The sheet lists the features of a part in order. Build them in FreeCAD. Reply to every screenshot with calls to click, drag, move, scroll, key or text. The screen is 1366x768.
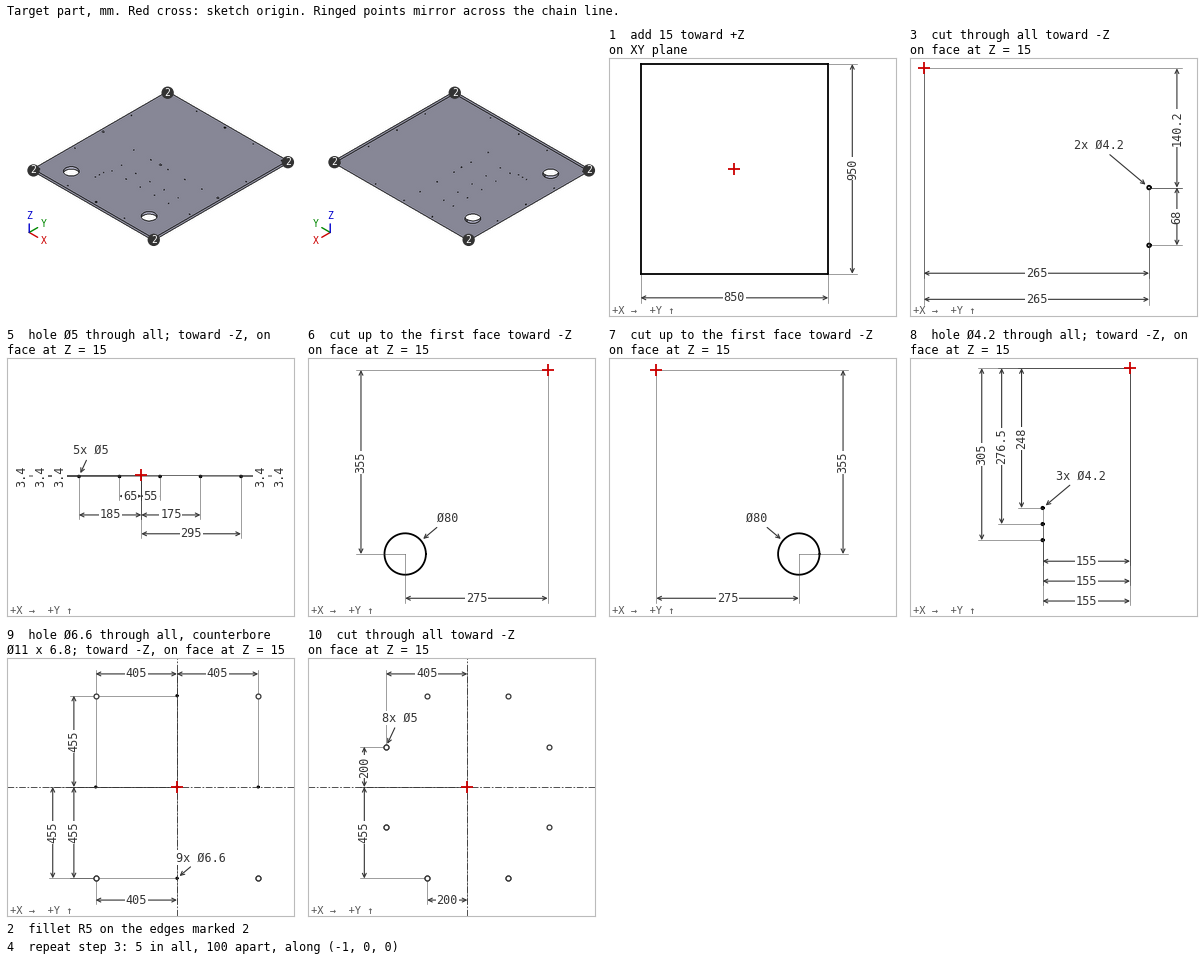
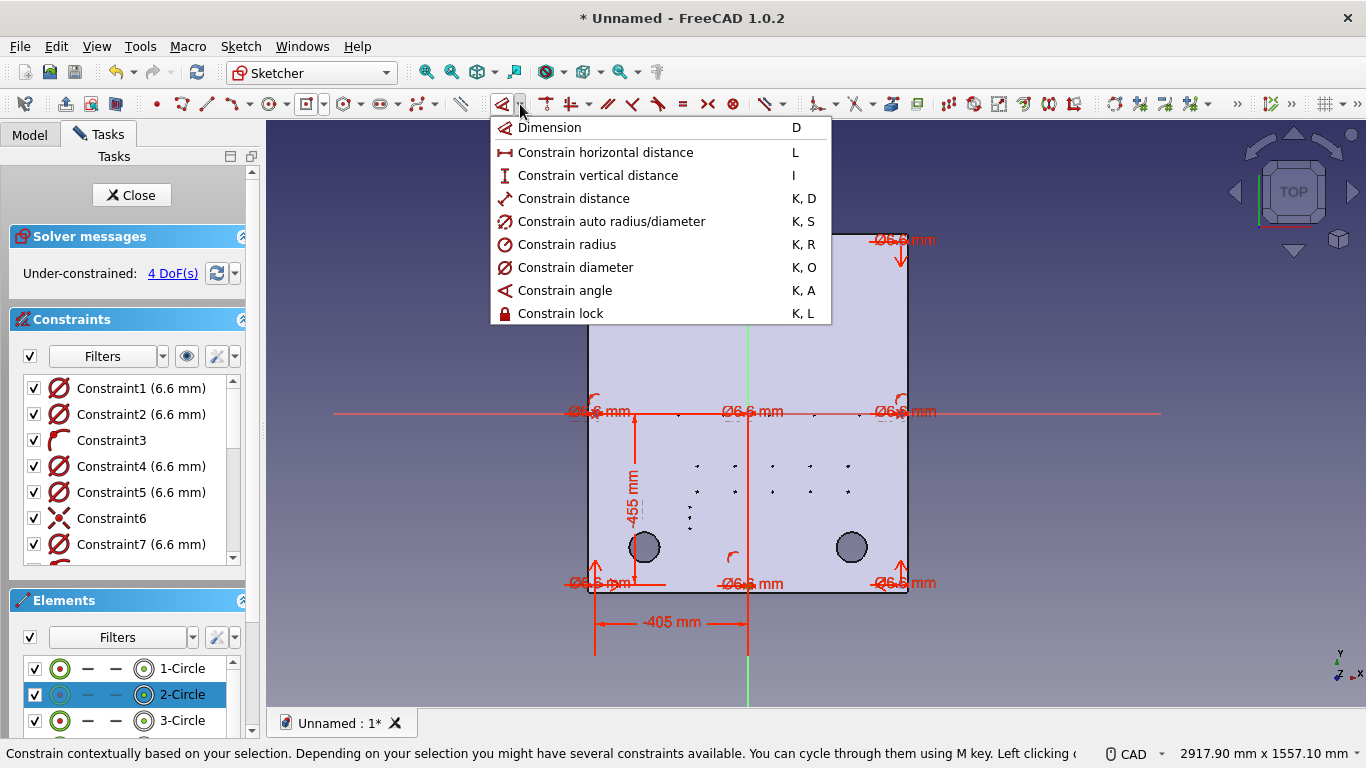
click(661, 176)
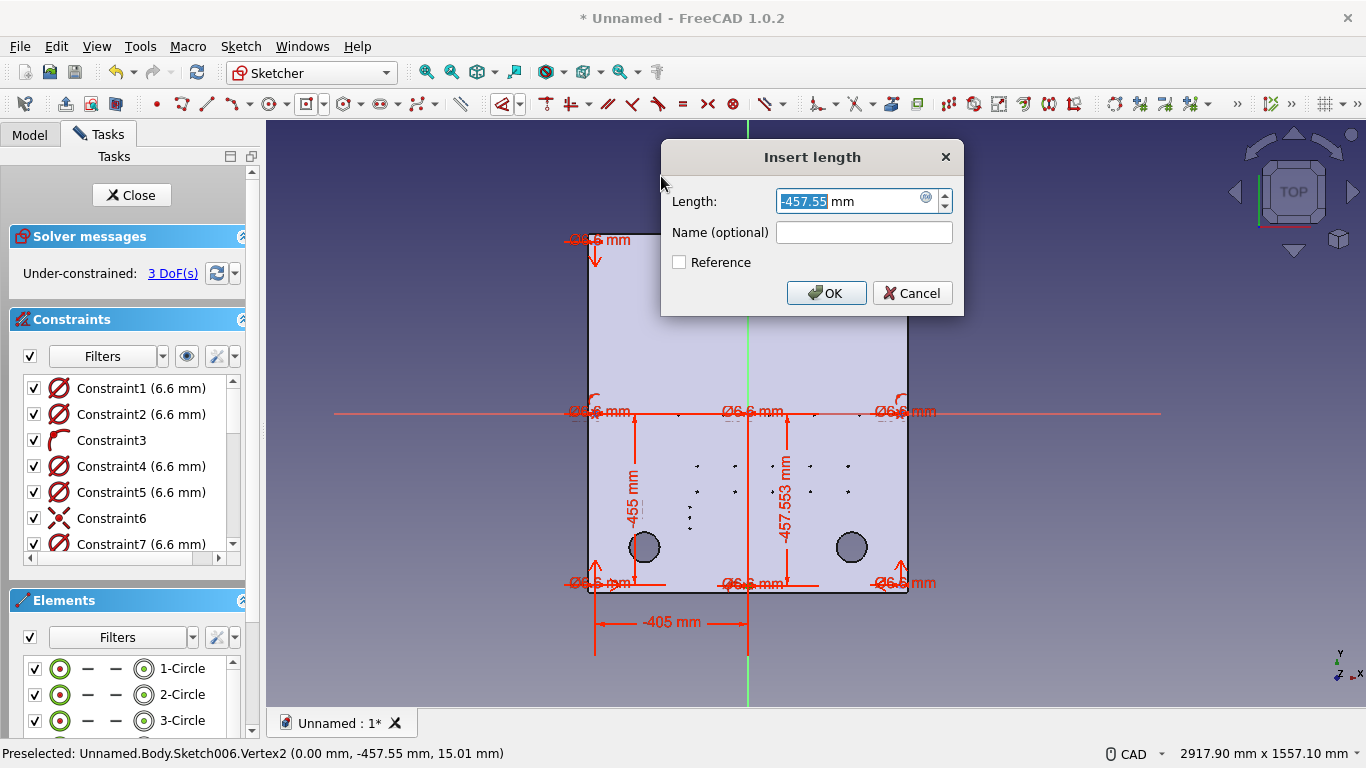
text(-455)
key(Return)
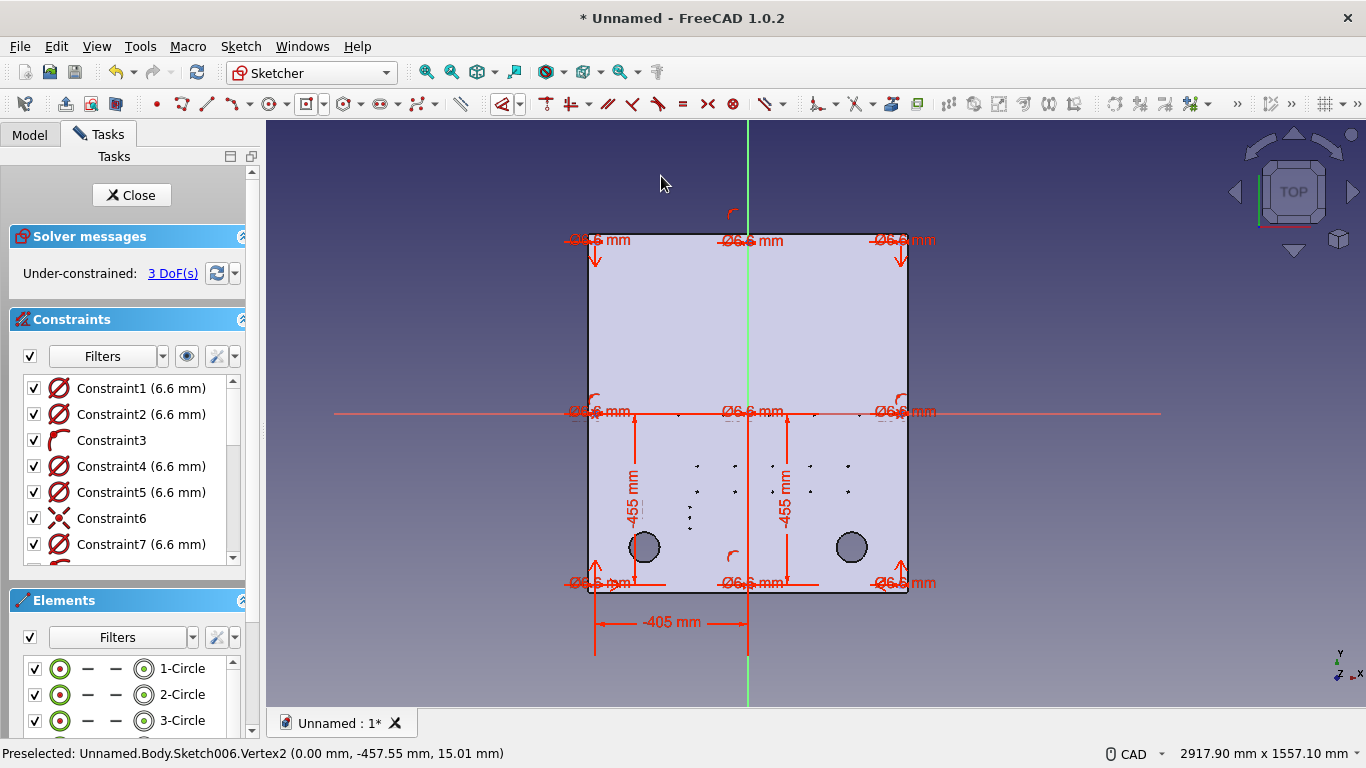
click(595, 414)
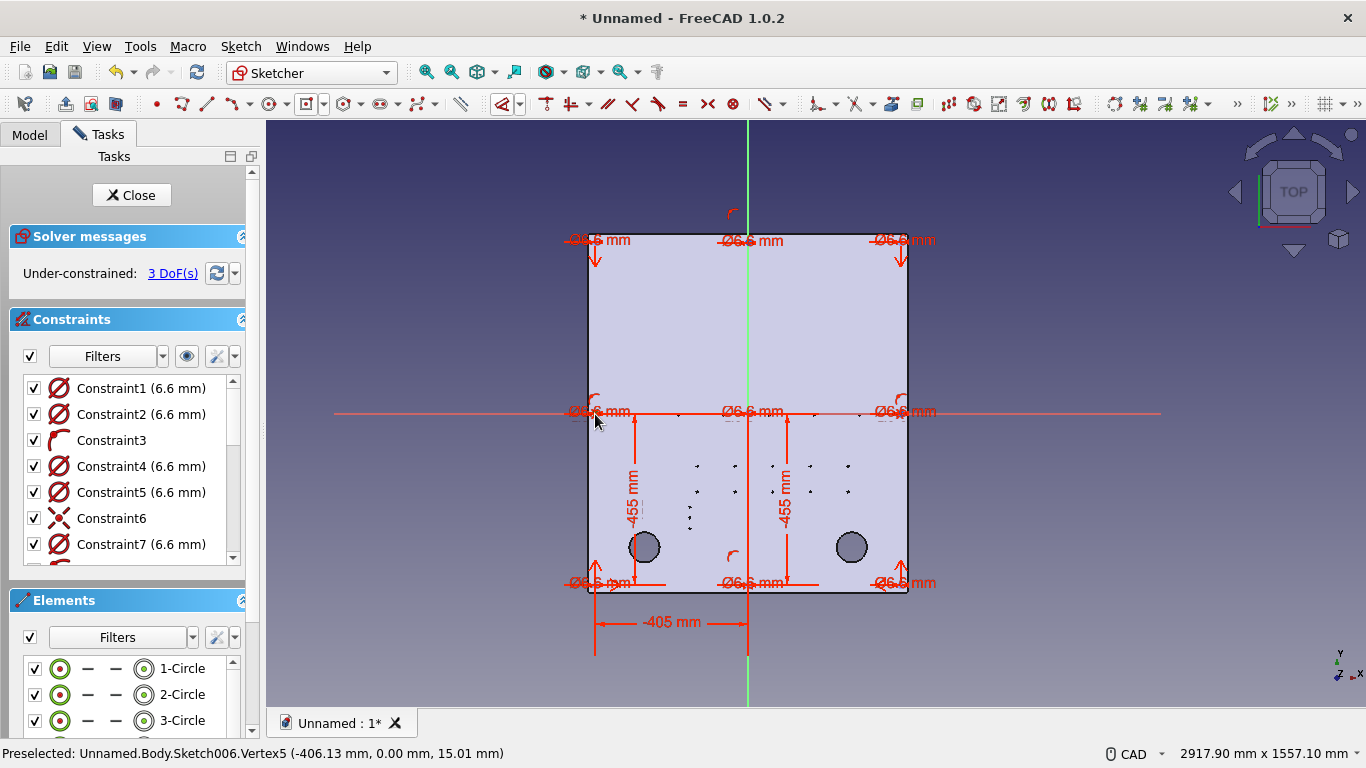
key(l)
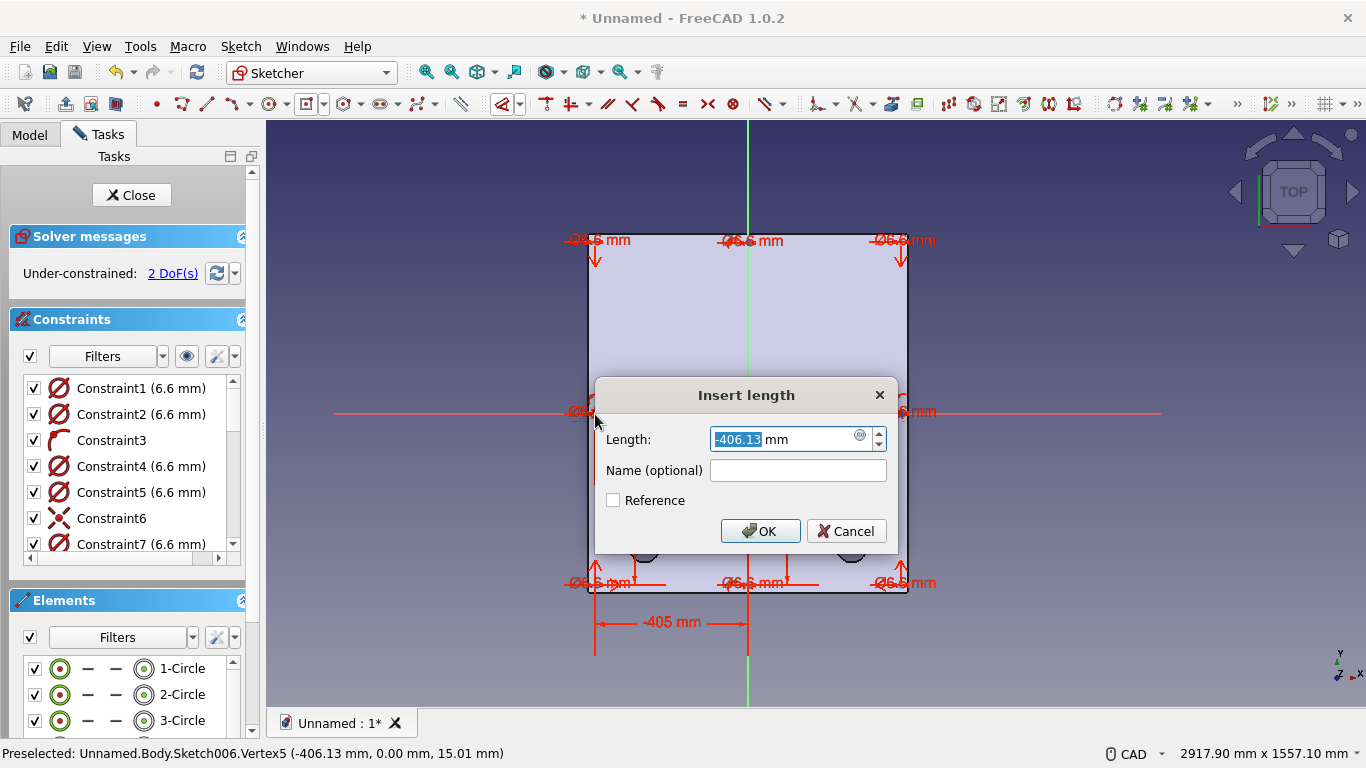
text(-405)
key(Return)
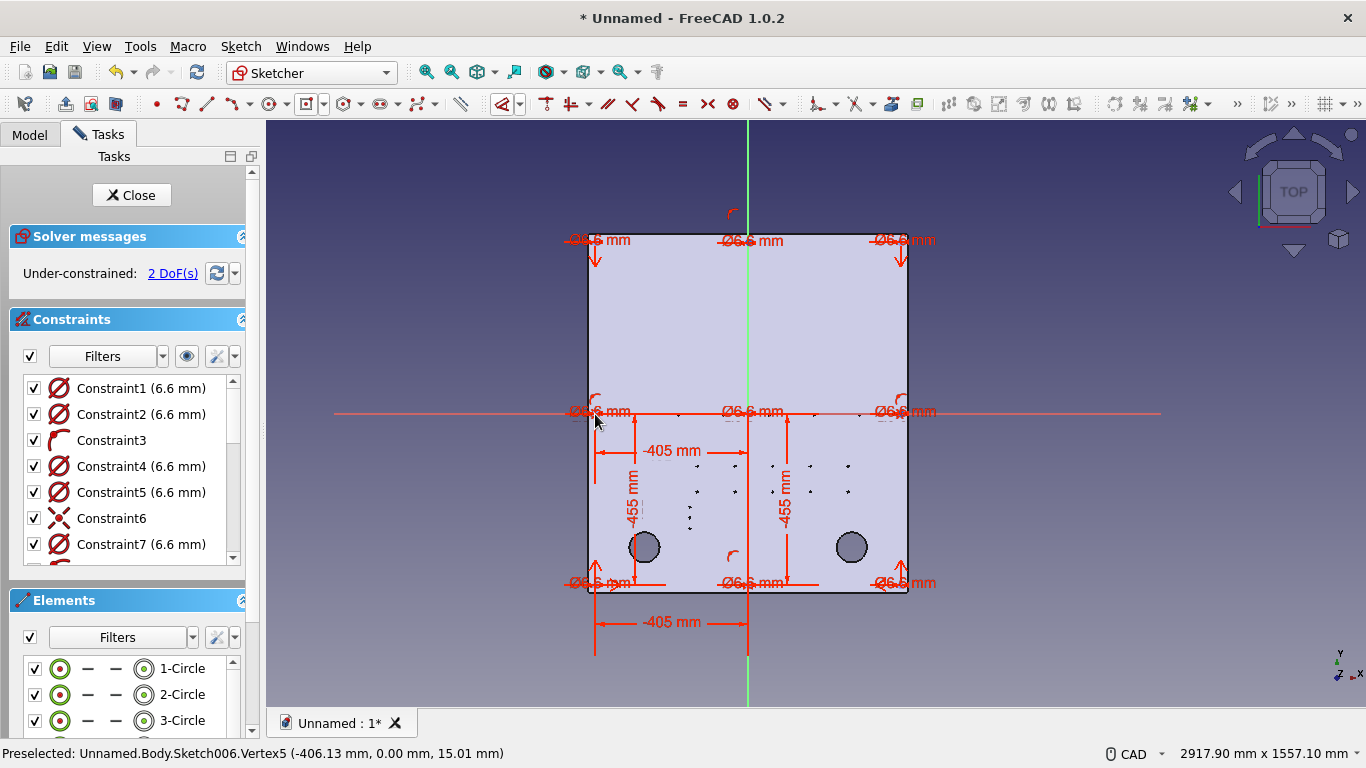
click(748, 243)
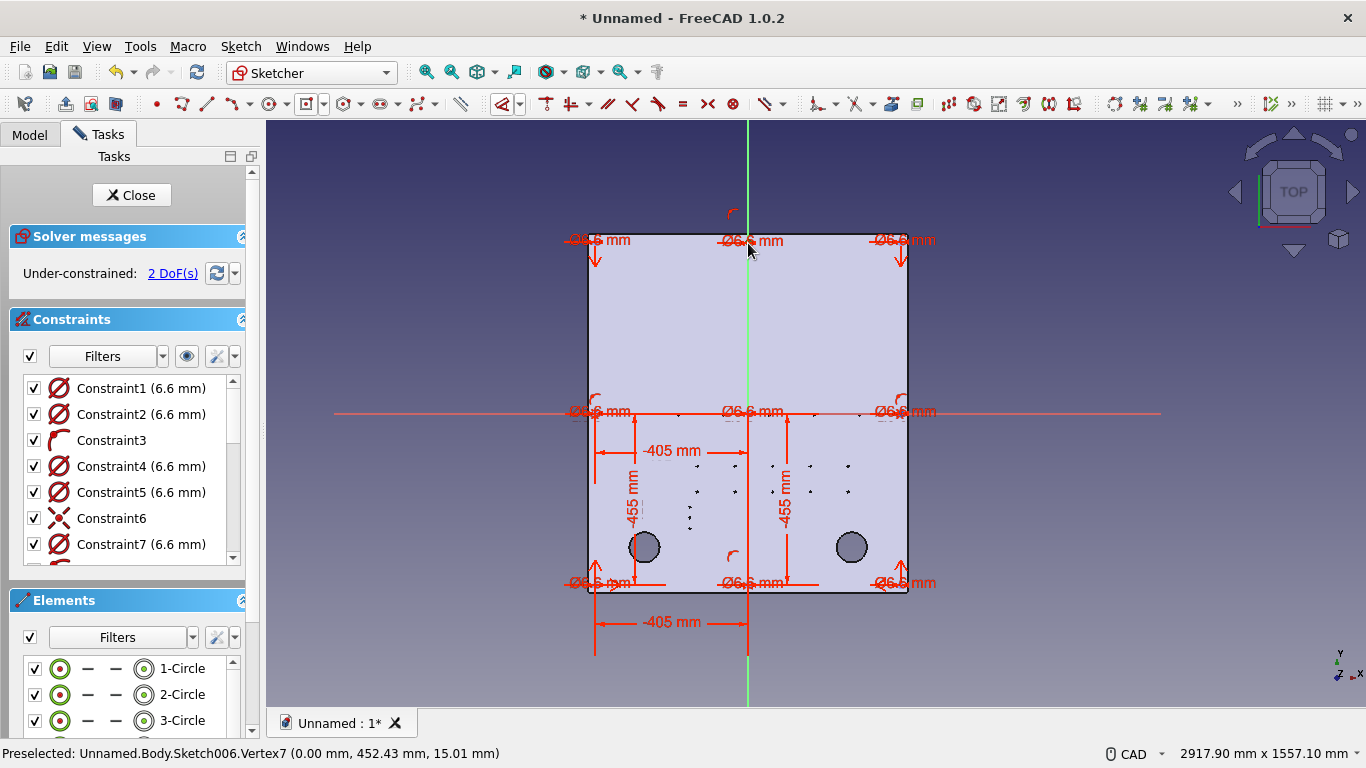
click(520, 104)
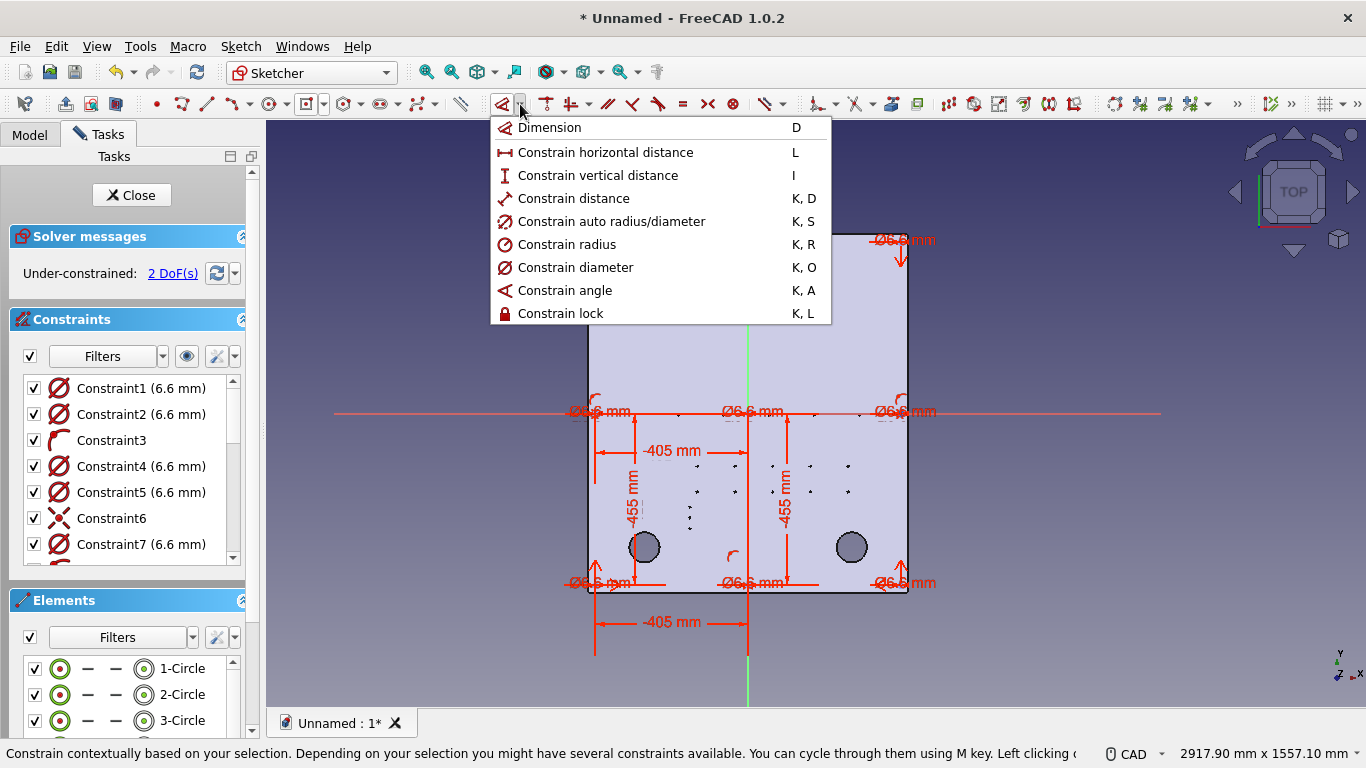
click(661, 176)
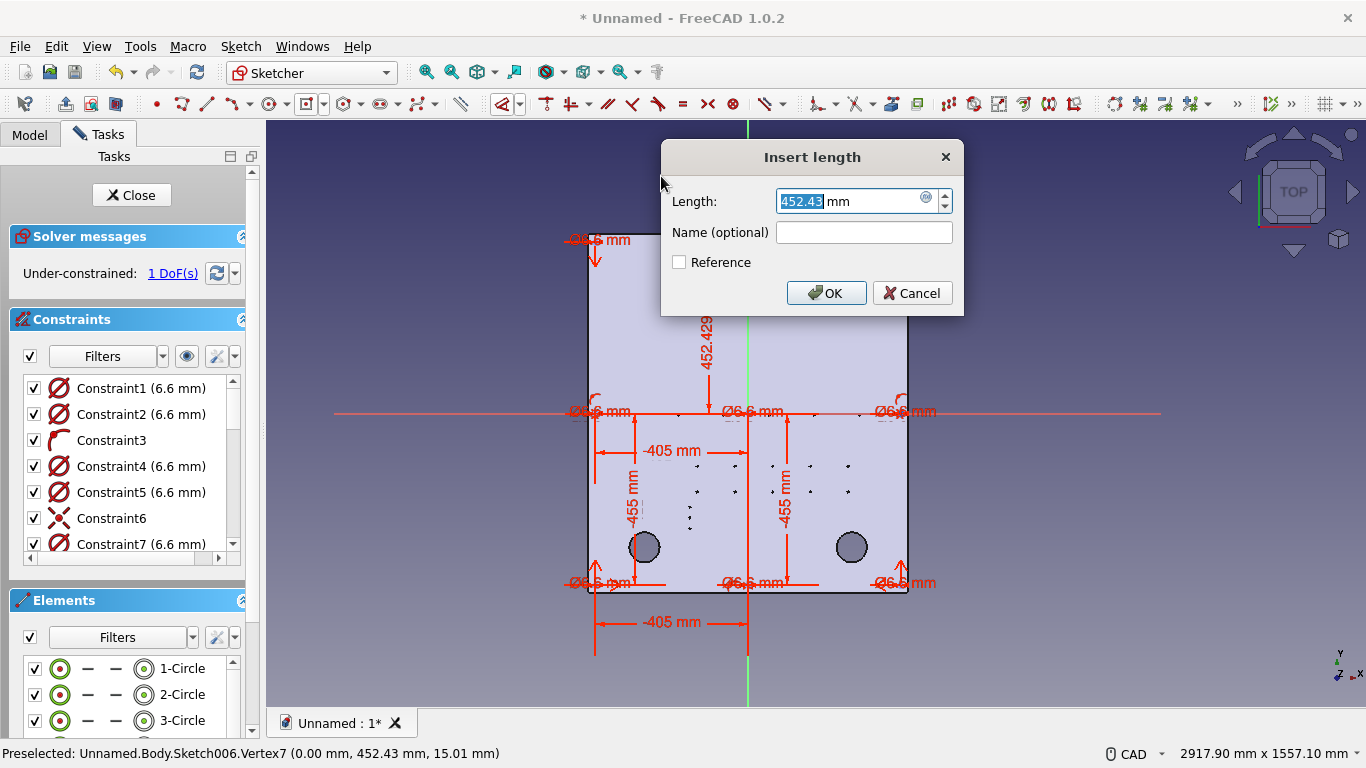
text(455)
key(Return)